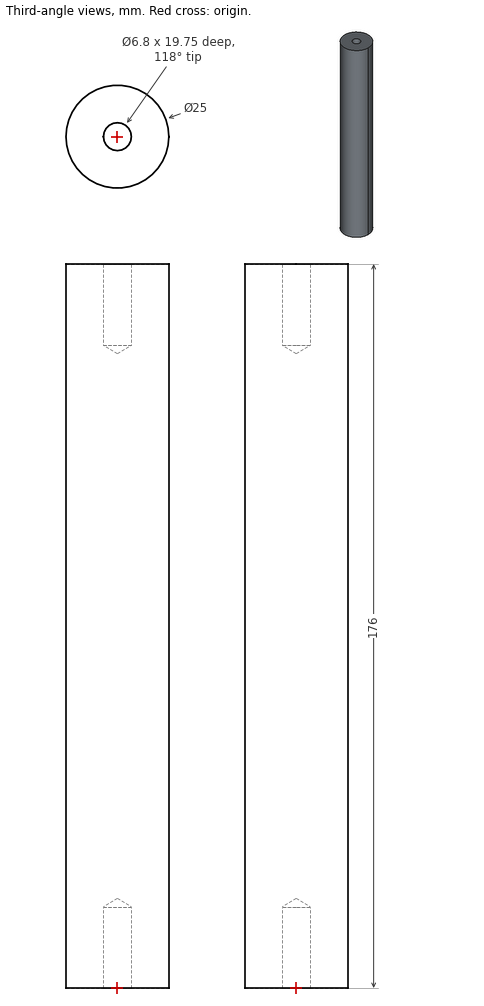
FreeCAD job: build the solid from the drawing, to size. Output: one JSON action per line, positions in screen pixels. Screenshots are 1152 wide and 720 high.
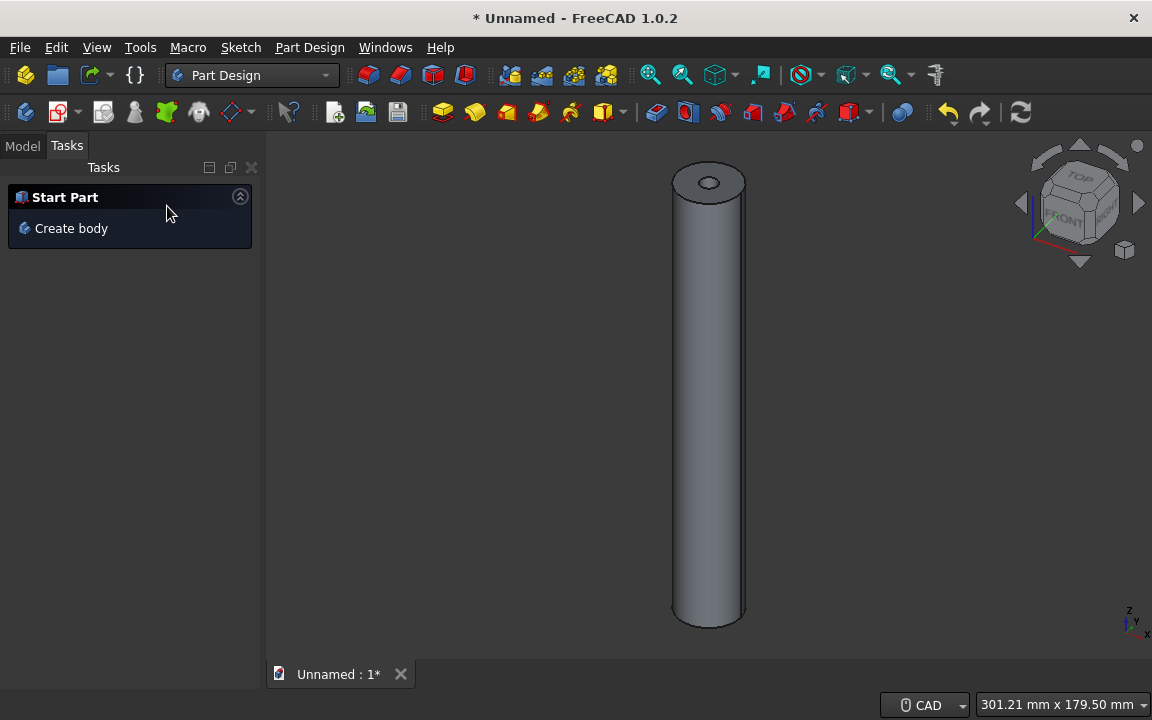
{"action": "key", "text": "0"}